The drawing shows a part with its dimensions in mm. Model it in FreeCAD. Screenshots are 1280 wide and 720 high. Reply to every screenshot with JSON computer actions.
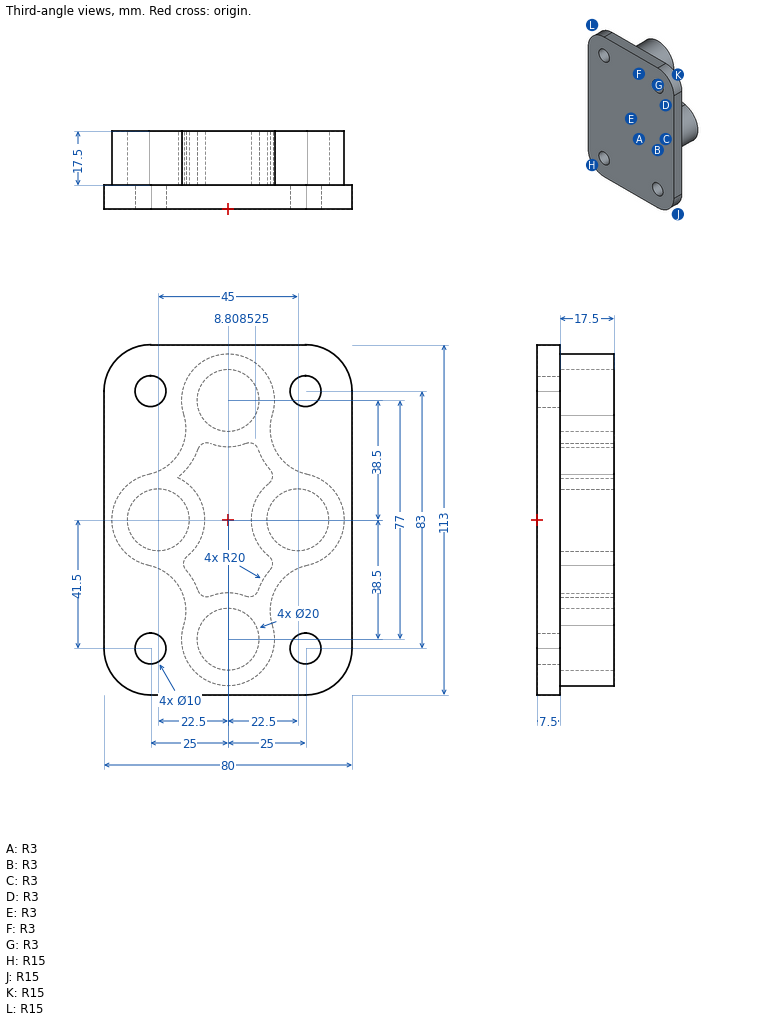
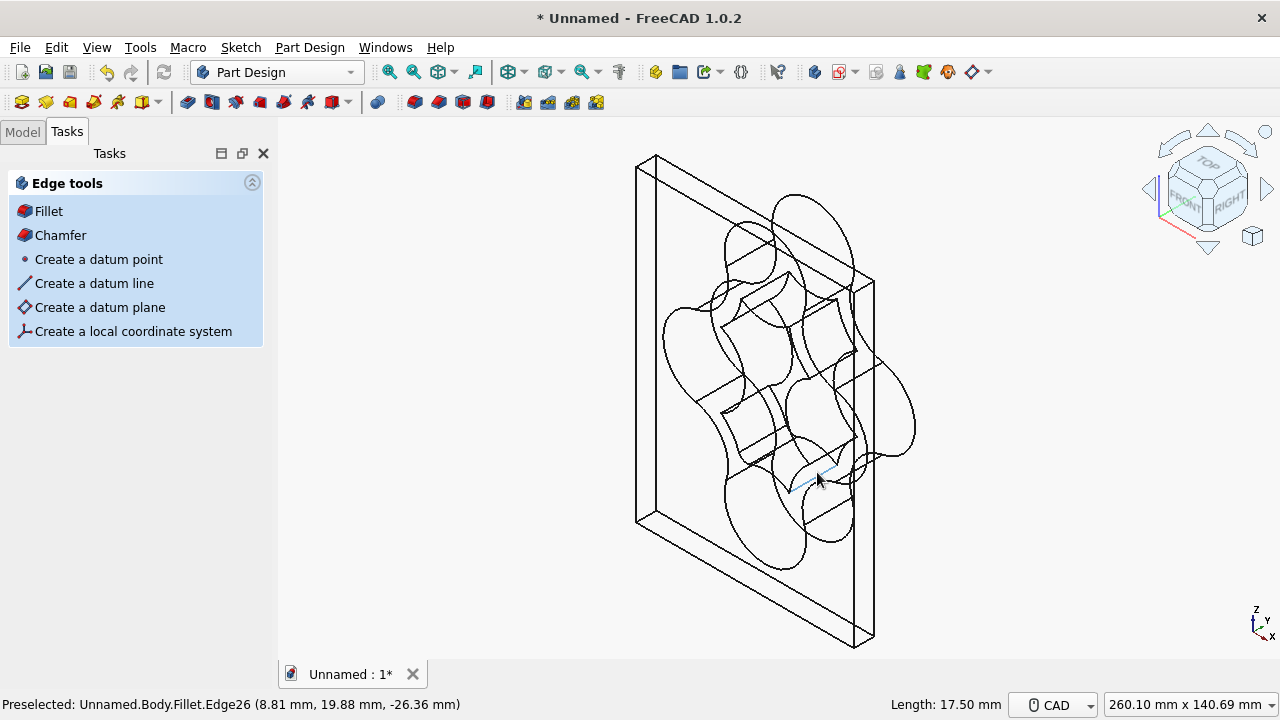
{"action": "key", "text": "v 1"}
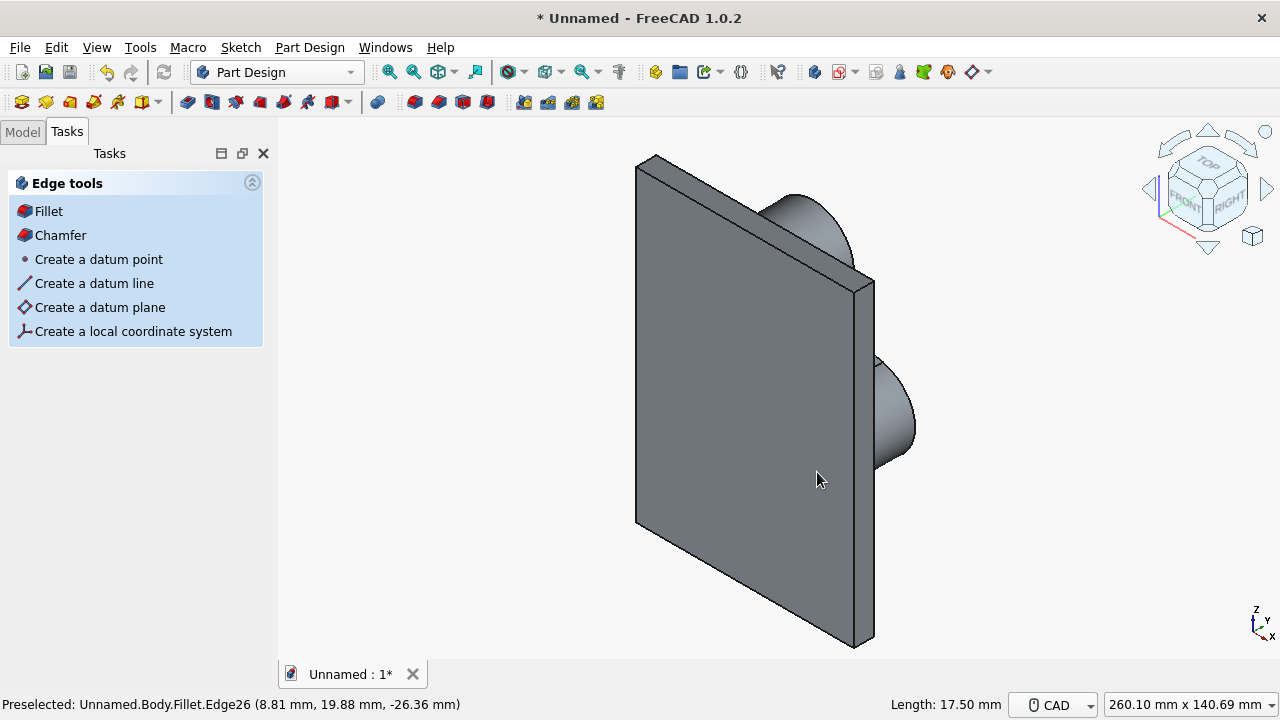
{"action": "left_click", "coordinate": [416, 102]}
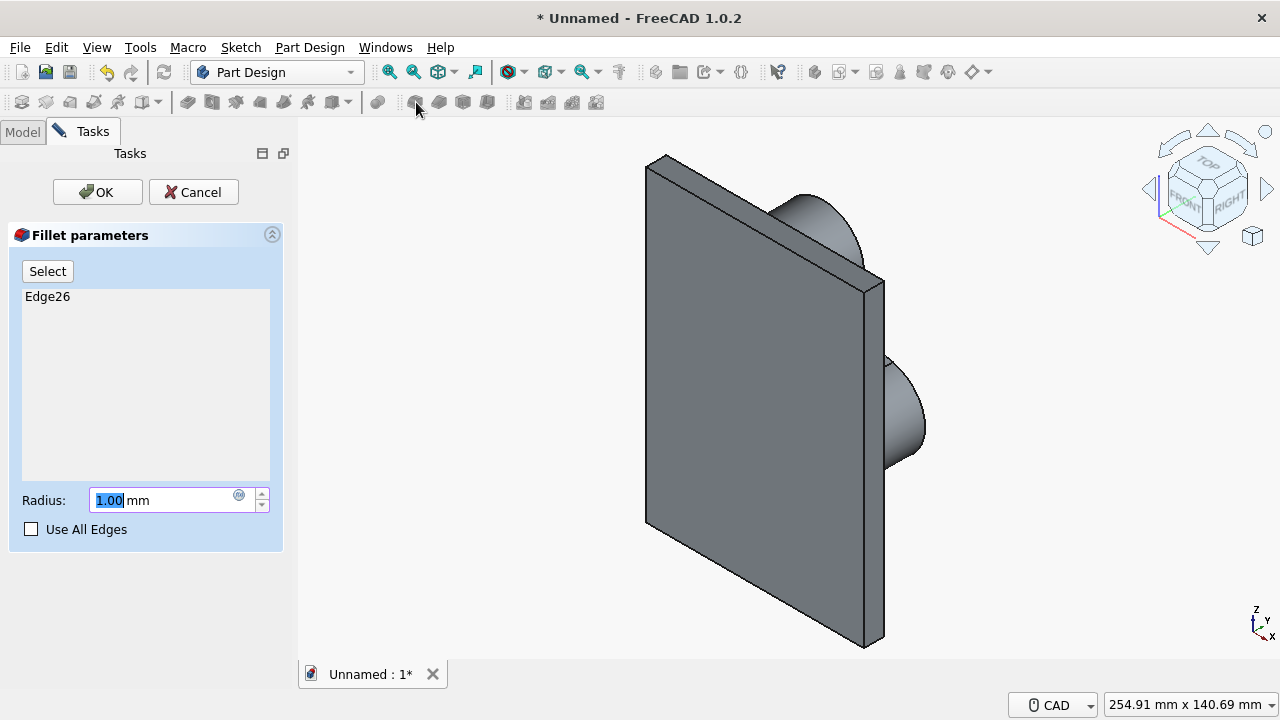
{"action": "type", "text": "3"}
{"action": "key", "text": "Tab"}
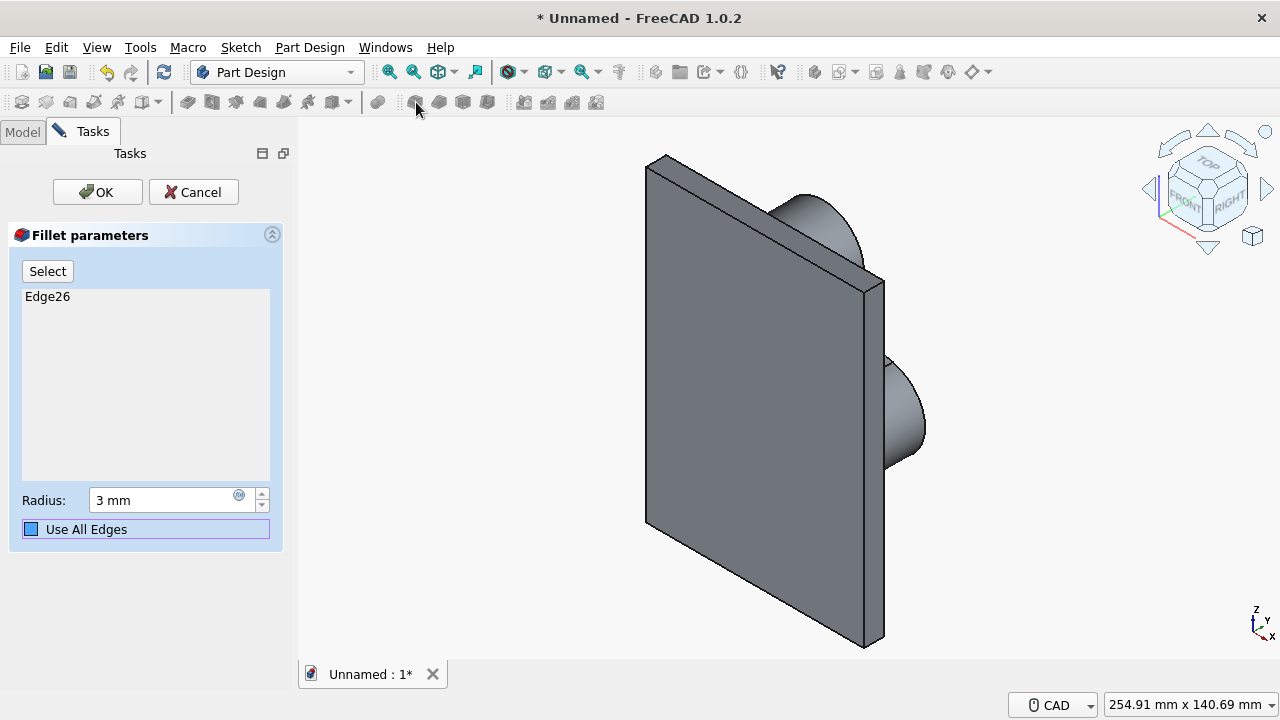
{"action": "left_click", "coordinate": [98, 192]}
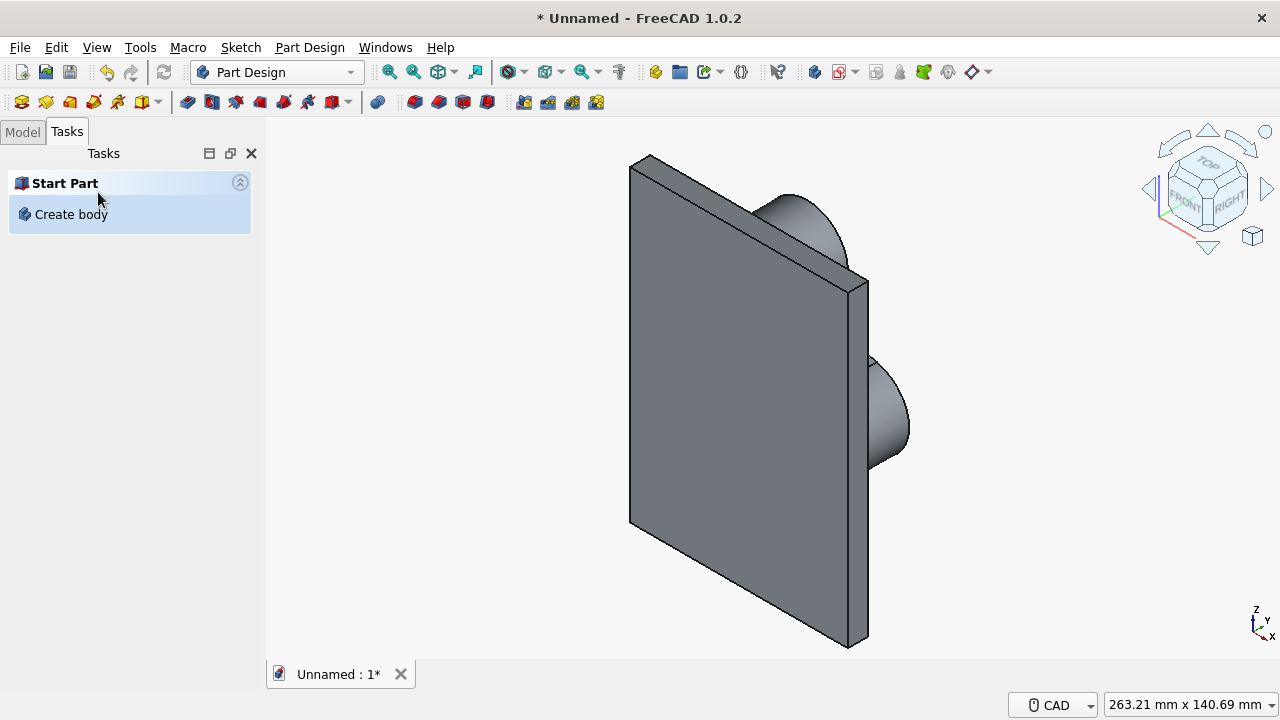
{"action": "key", "text": "2"}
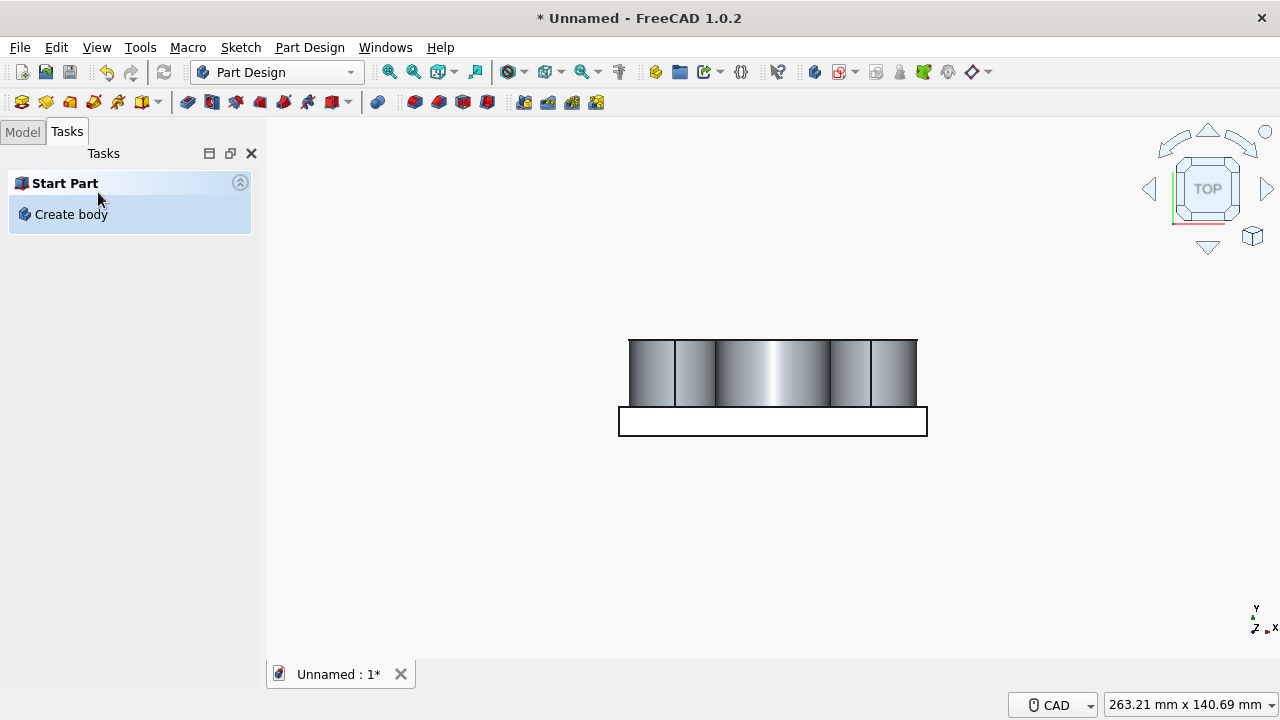
{"action": "key", "text": "v f"}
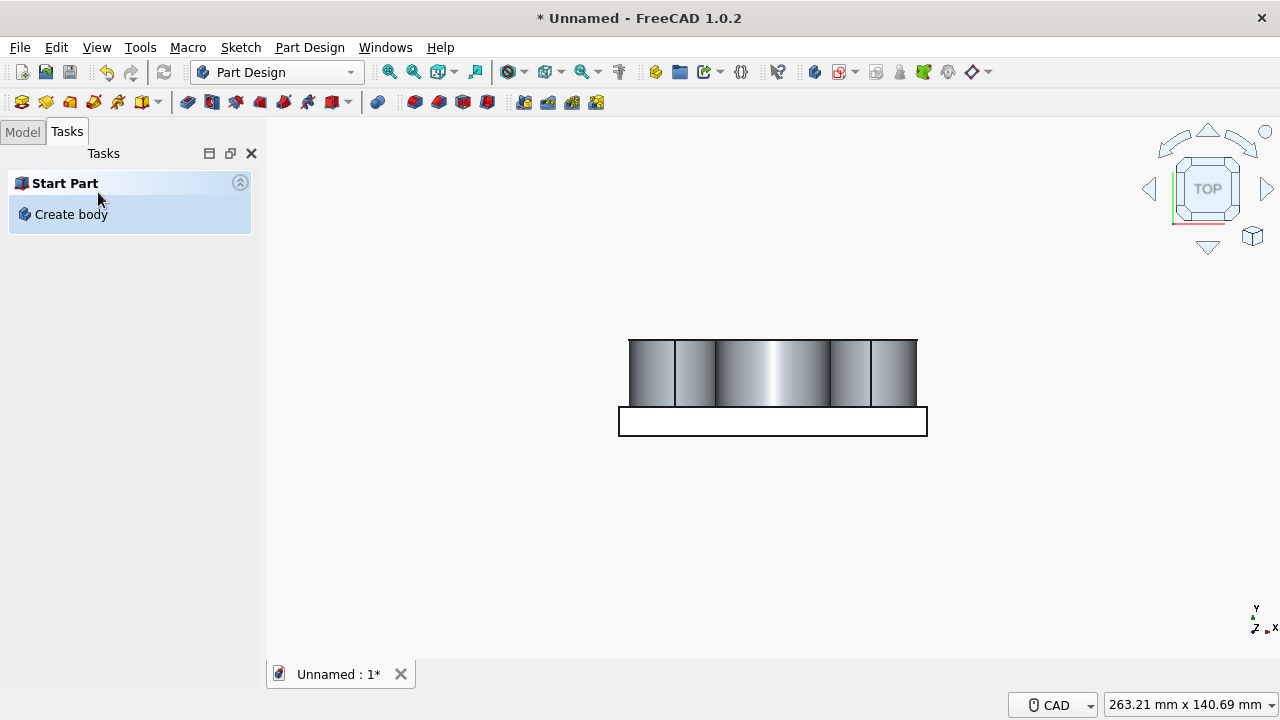
{"action": "key", "text": "0"}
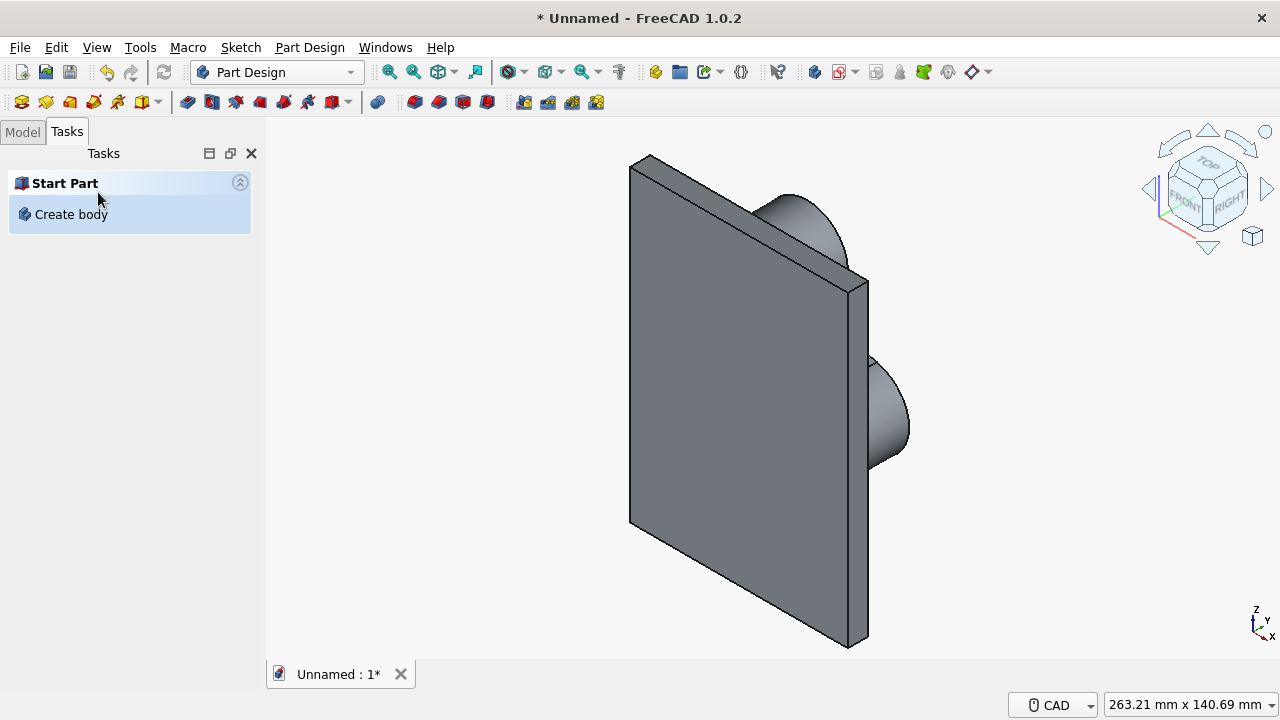
{"action": "key", "text": "1"}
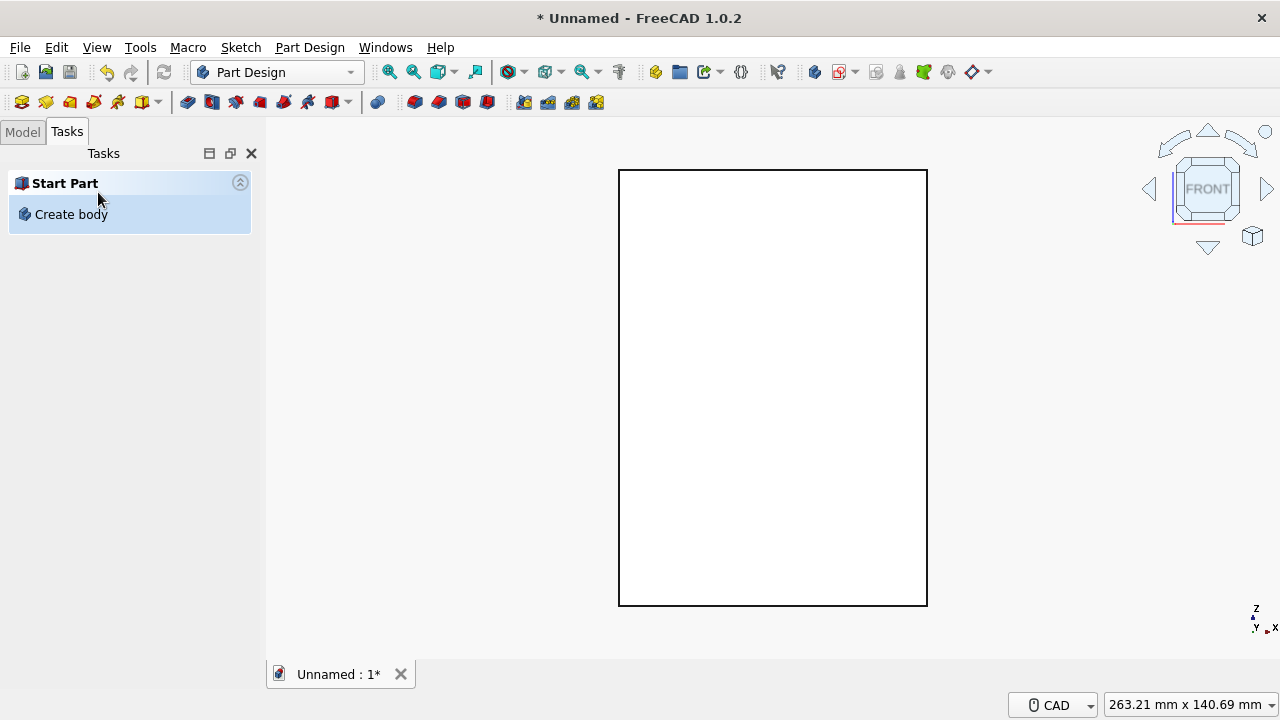
{"action": "key", "text": "3"}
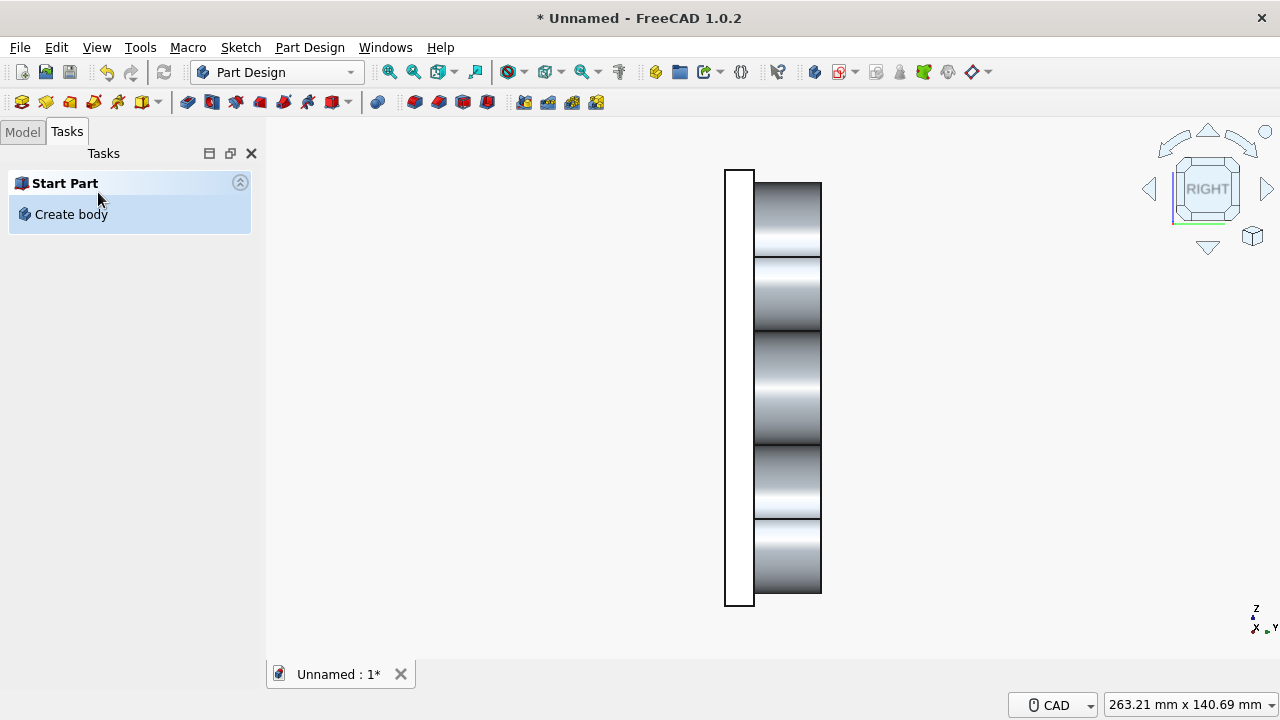
{"action": "key", "text": "5"}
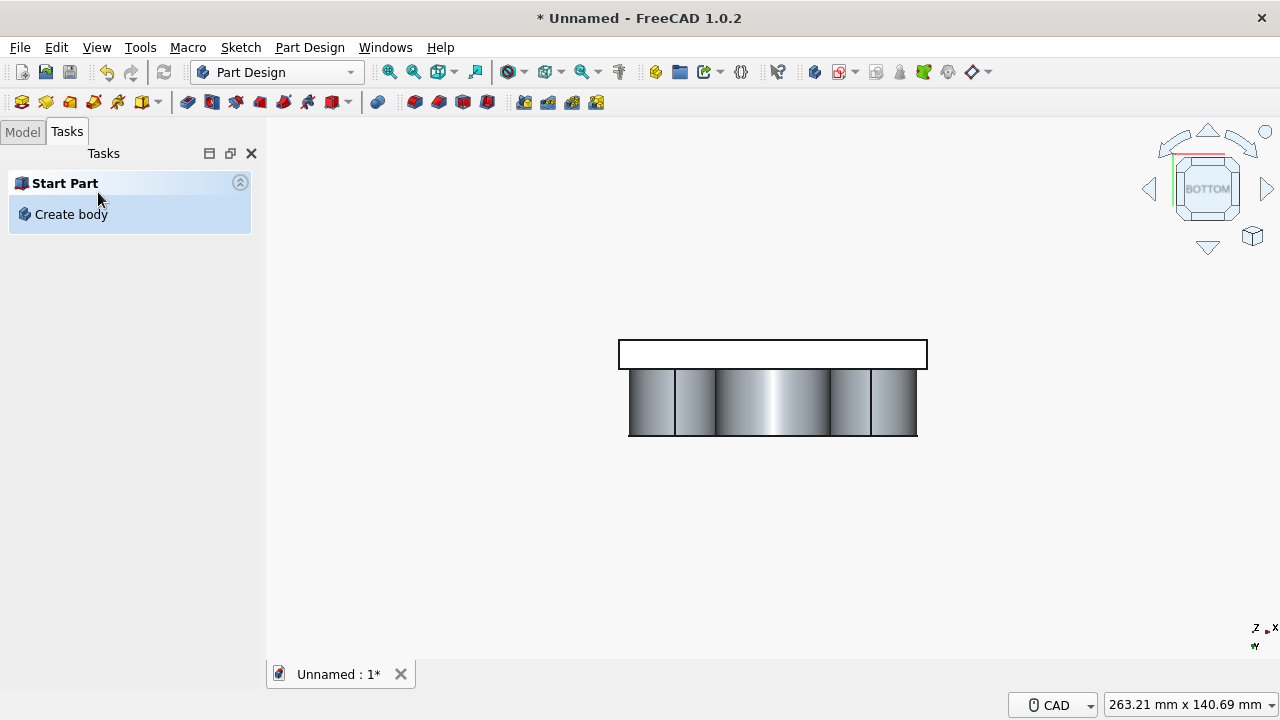
{"action": "key", "text": "v f"}